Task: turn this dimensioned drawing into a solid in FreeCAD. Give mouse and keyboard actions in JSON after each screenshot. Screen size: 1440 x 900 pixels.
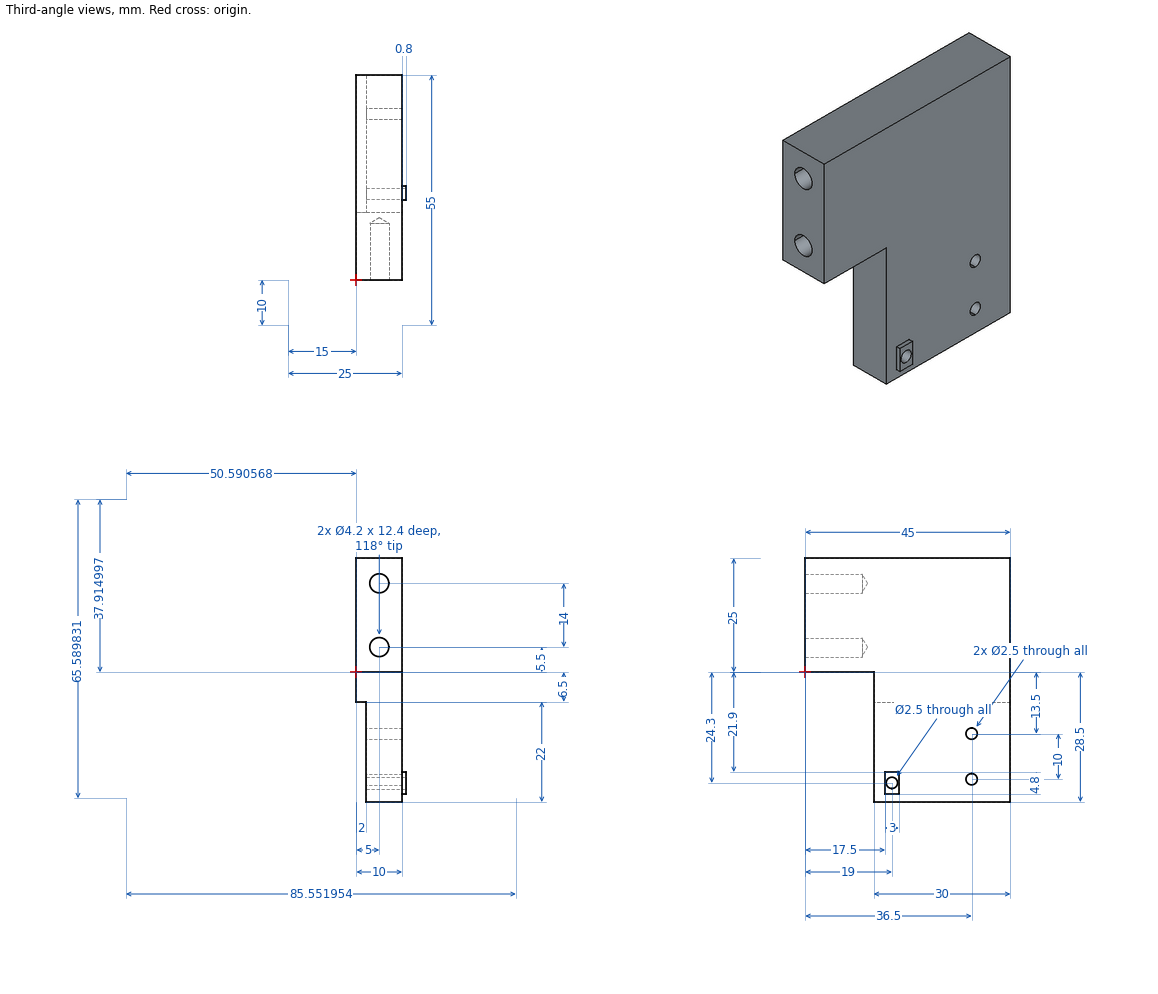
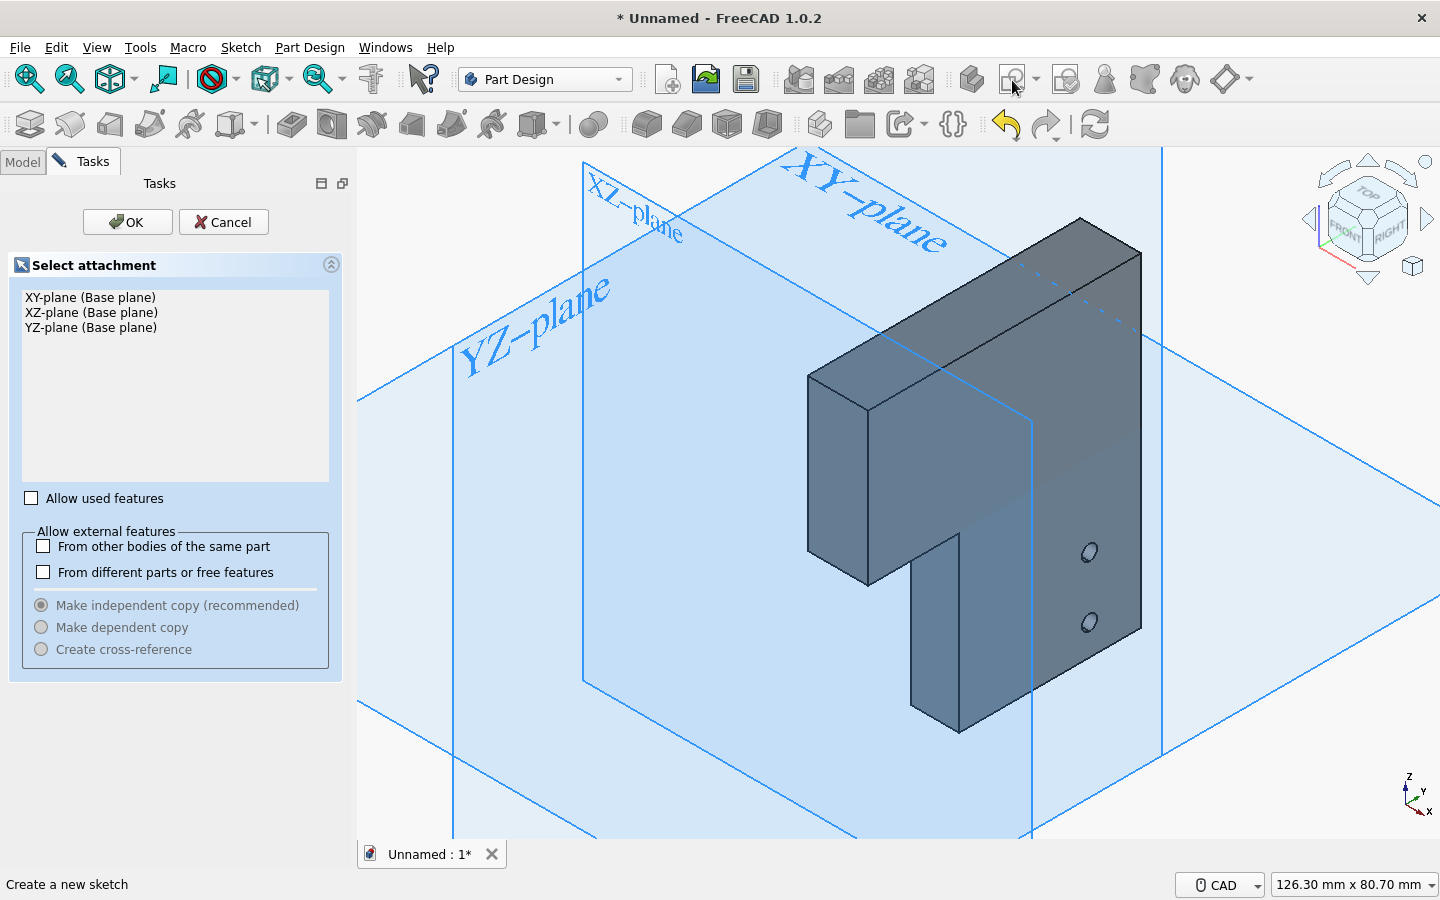
{"action": "left_click", "coordinate": [82, 312]}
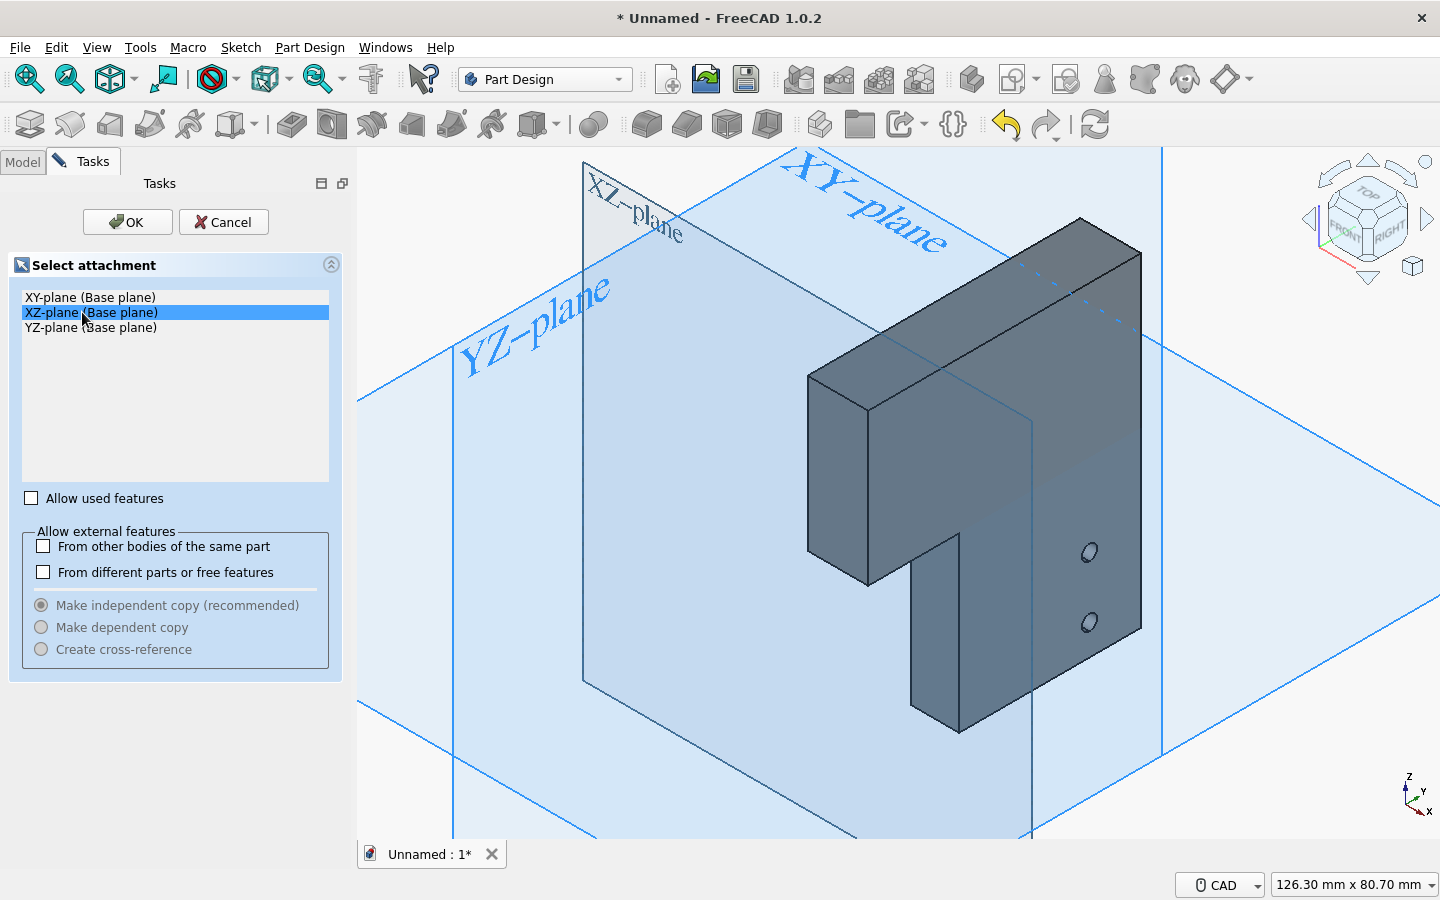
{"action": "left_click", "coordinate": [128, 222]}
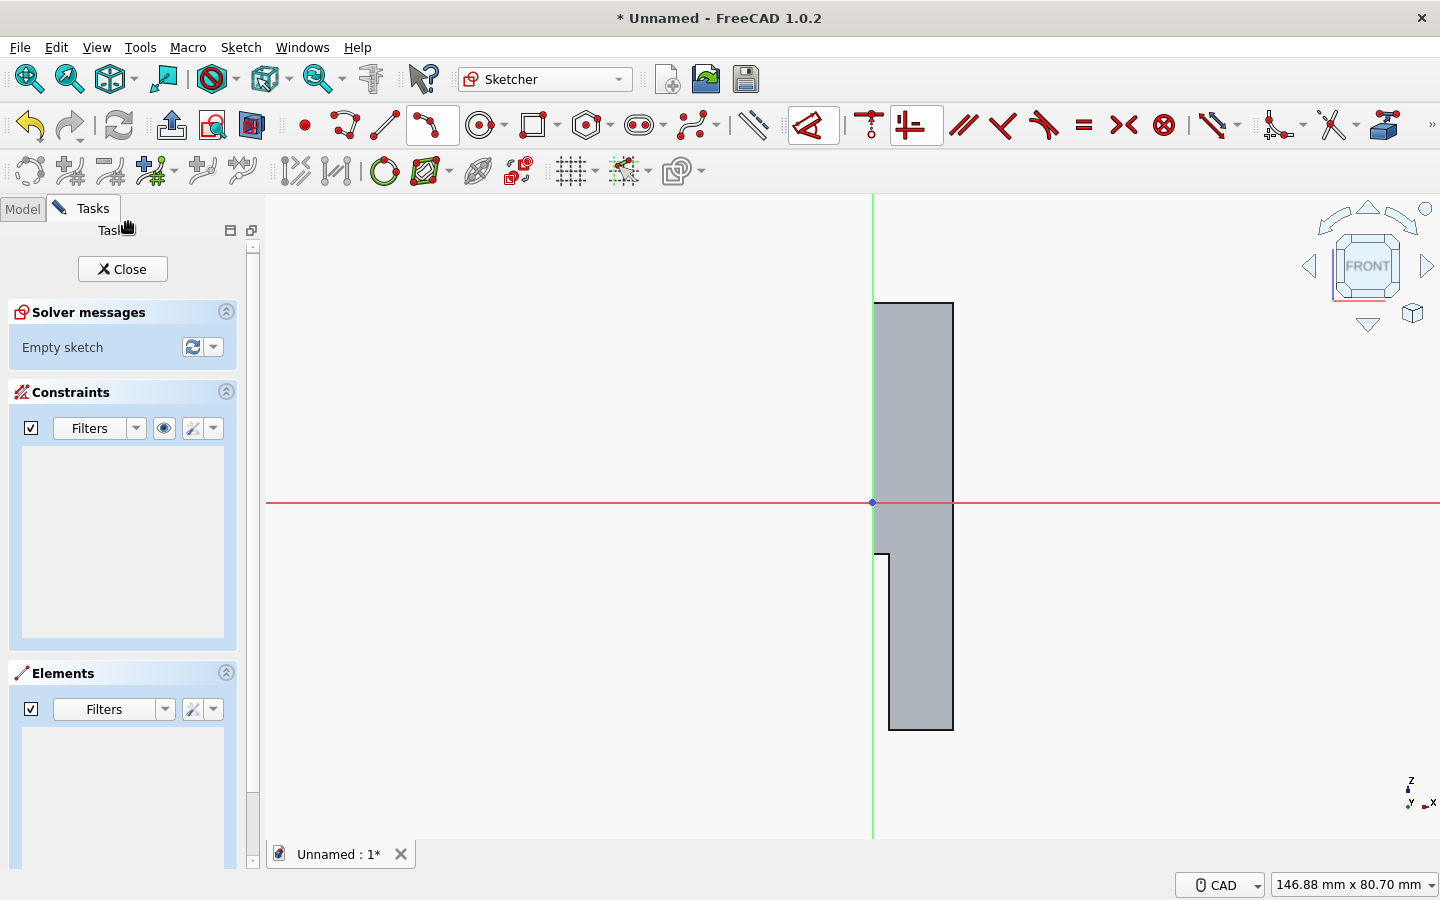
{"action": "scroll", "coordinate": [997, 334], "scroll_direction": "up", "scroll_amount": 4}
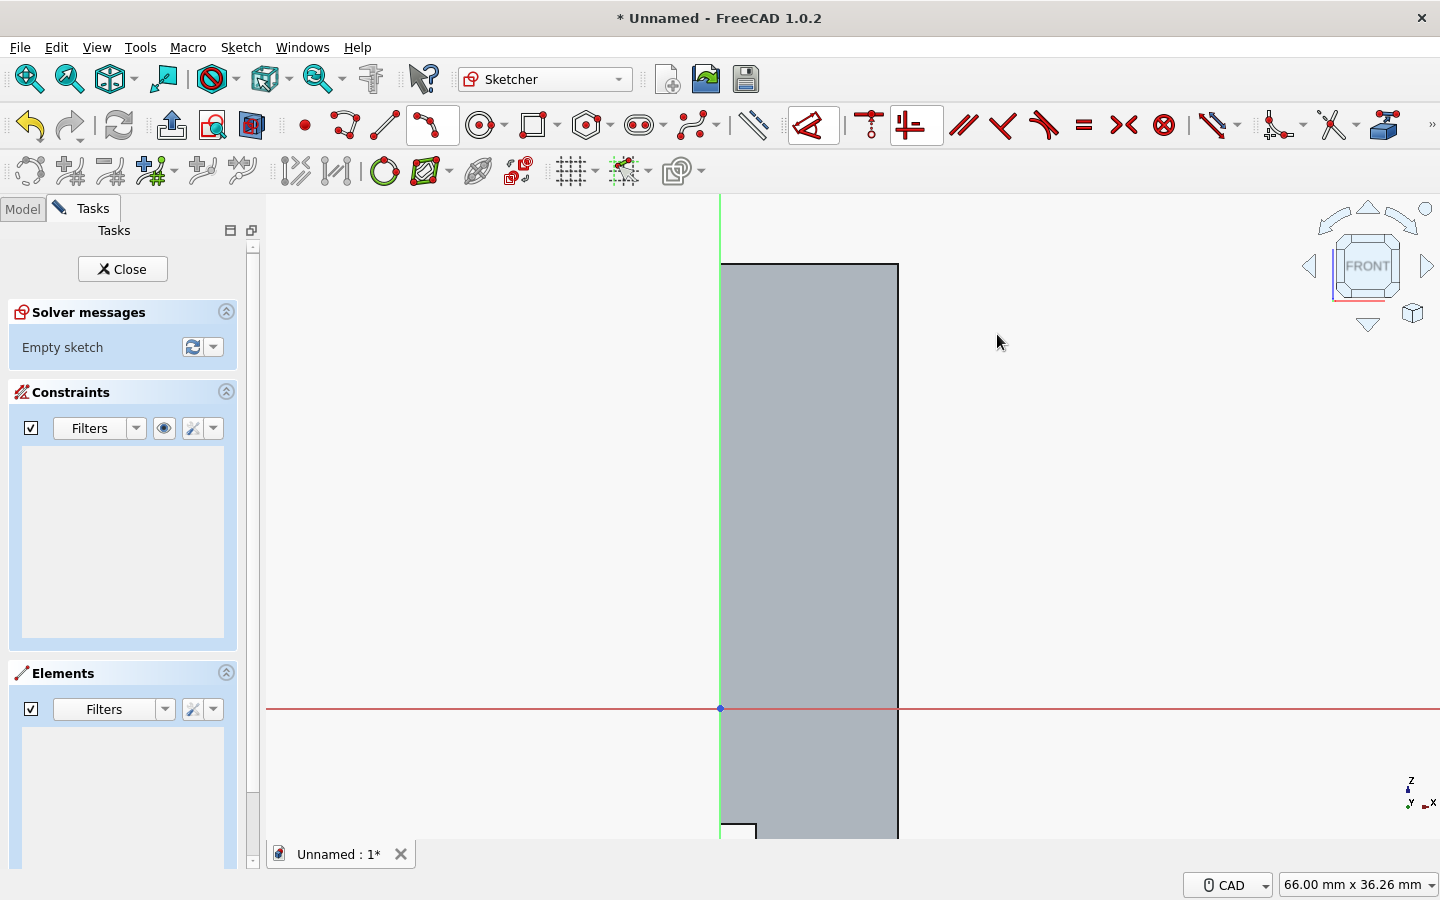
{"action": "key", "text": "g c"}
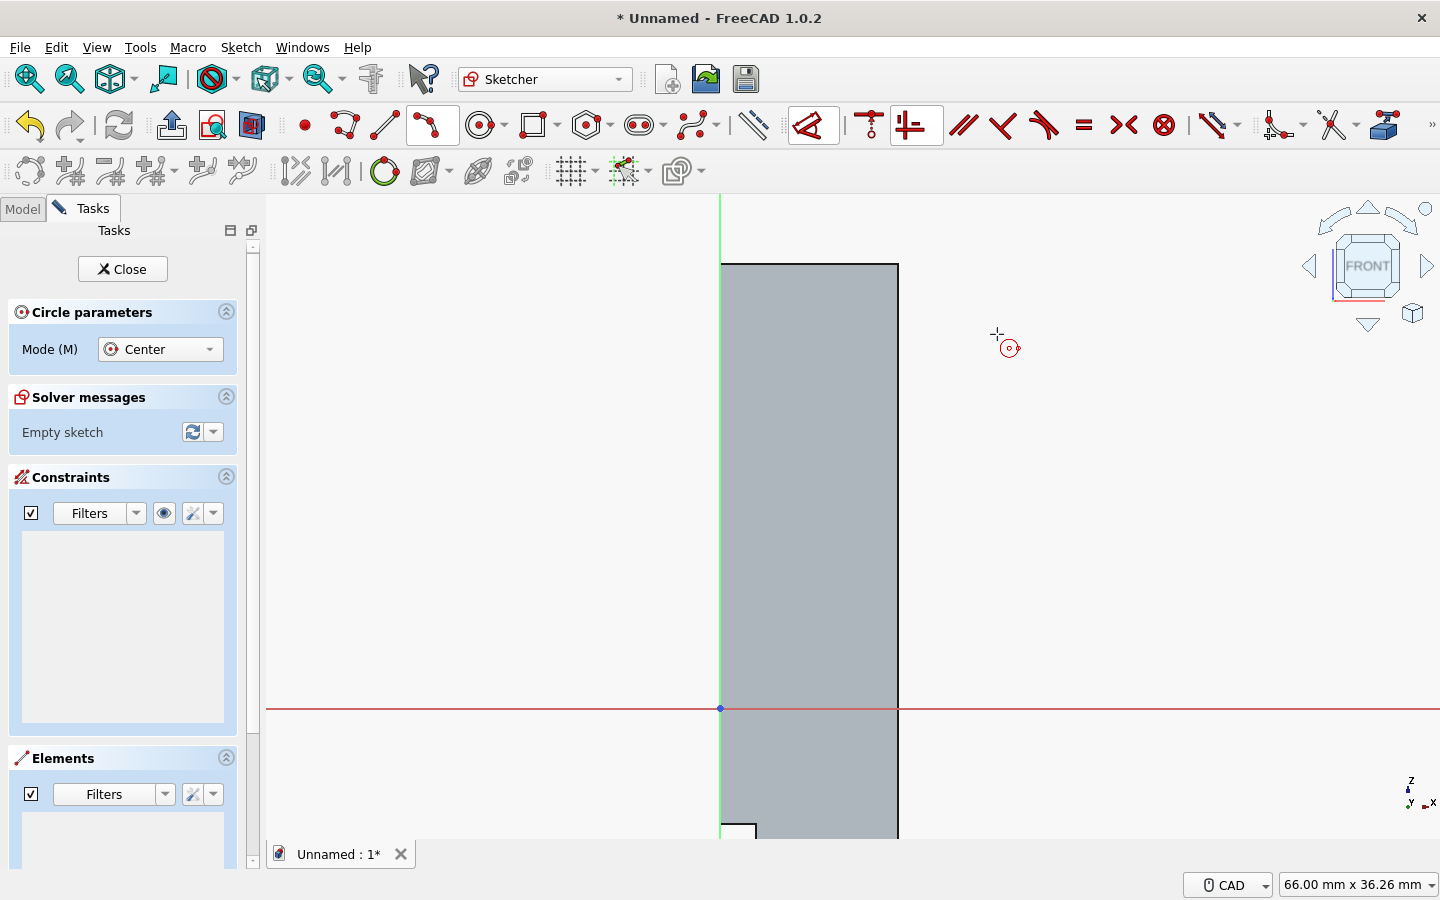
{"action": "left_click", "coordinate": [809, 611]}
{"action": "left_click", "coordinate": [836, 585]}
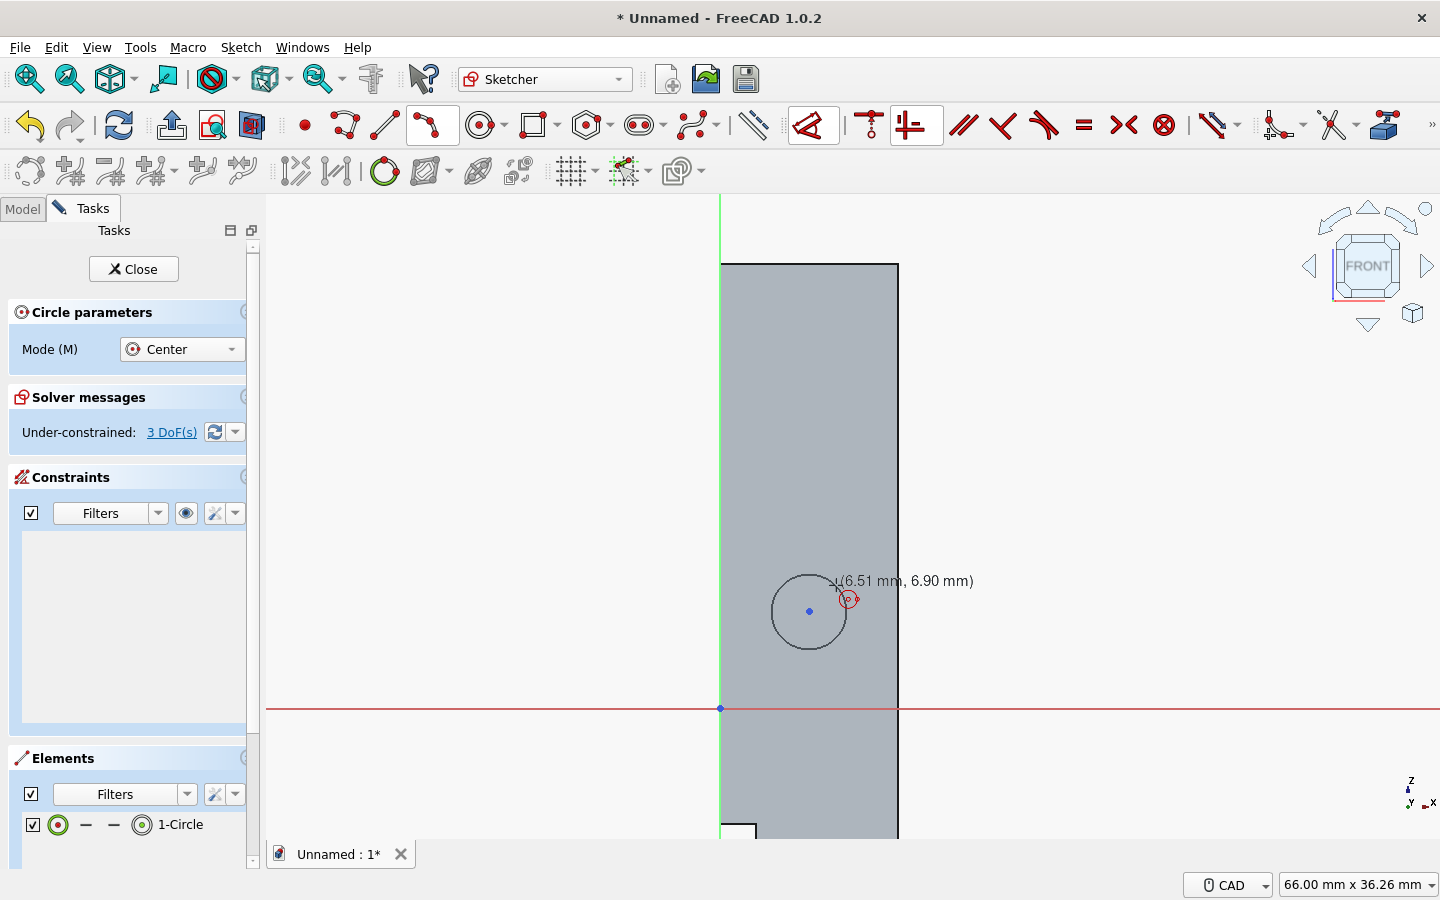
{"action": "left_click", "coordinate": [809, 362]}
{"action": "left_click", "coordinate": [836, 335]}
{"action": "key", "text": "Escape"}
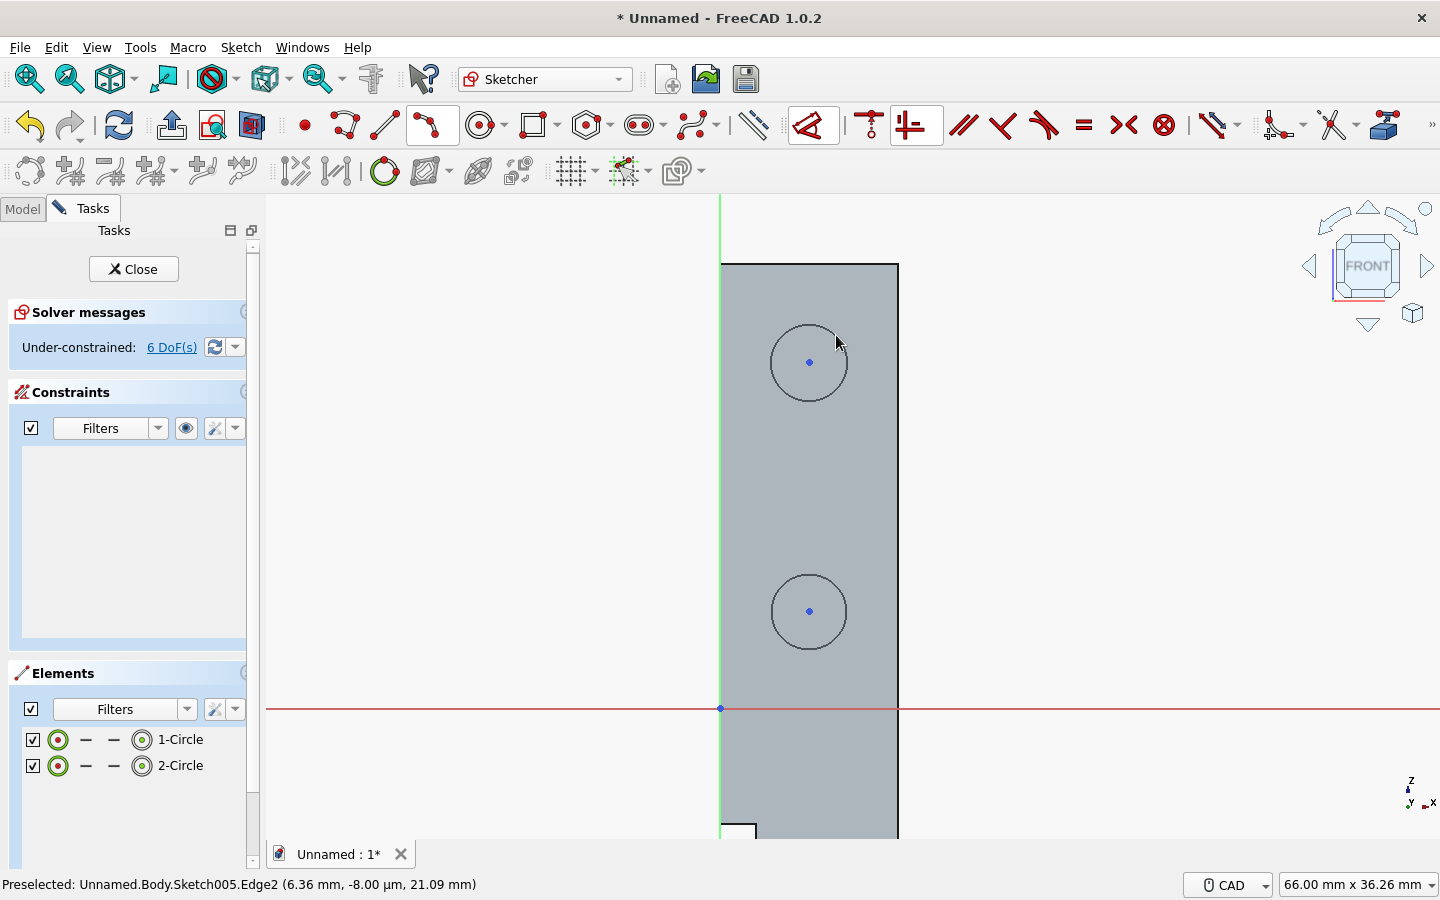
{"action": "left_click", "coordinate": [835, 585]}